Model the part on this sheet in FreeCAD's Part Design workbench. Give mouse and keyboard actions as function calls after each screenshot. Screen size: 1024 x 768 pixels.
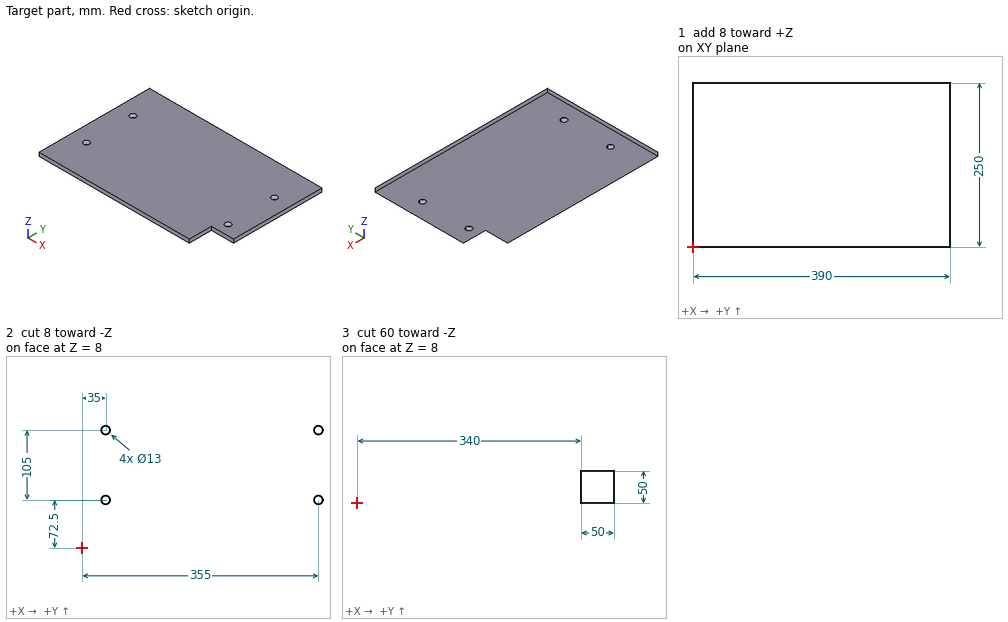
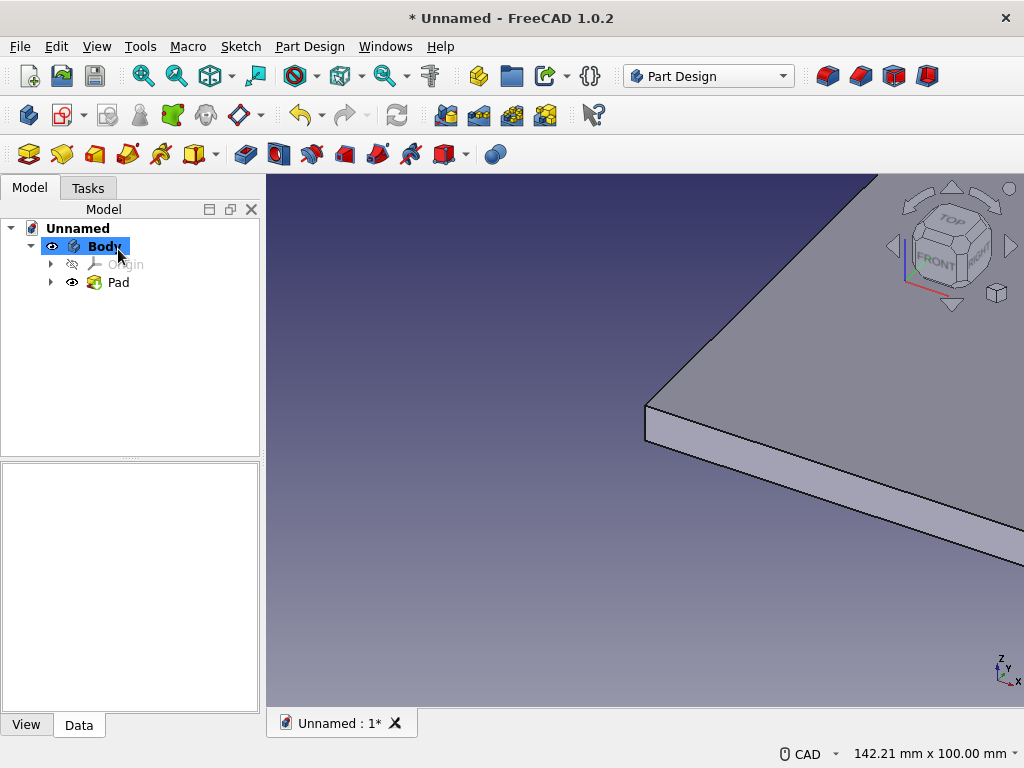
click(144, 76)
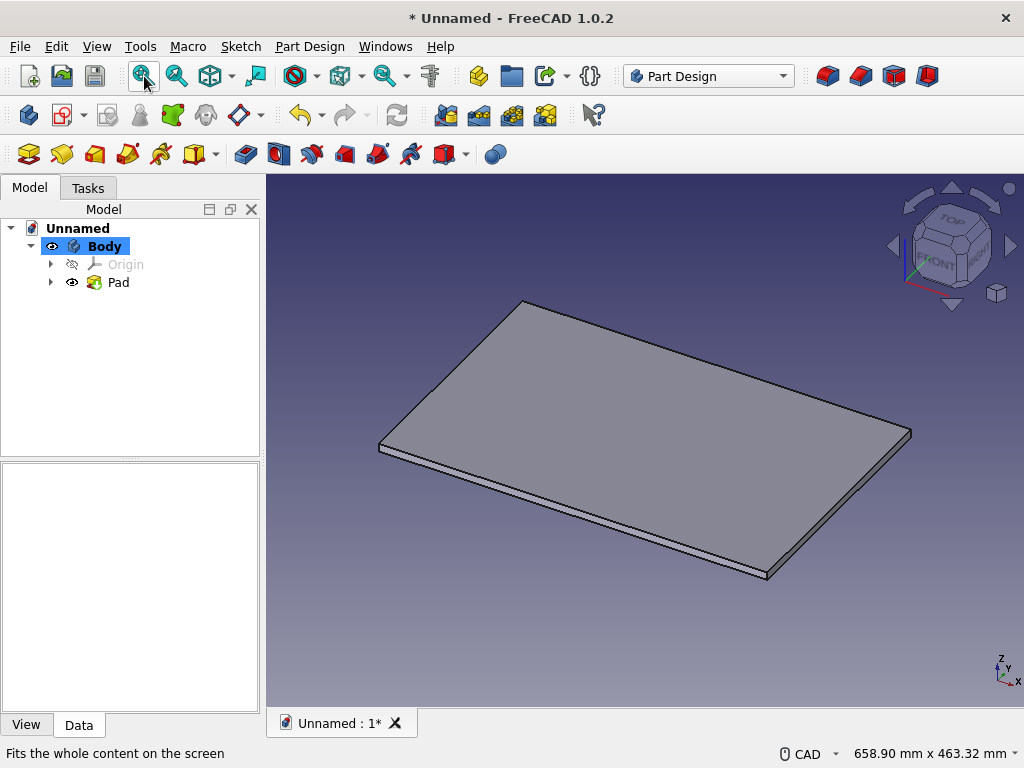
click(701, 454)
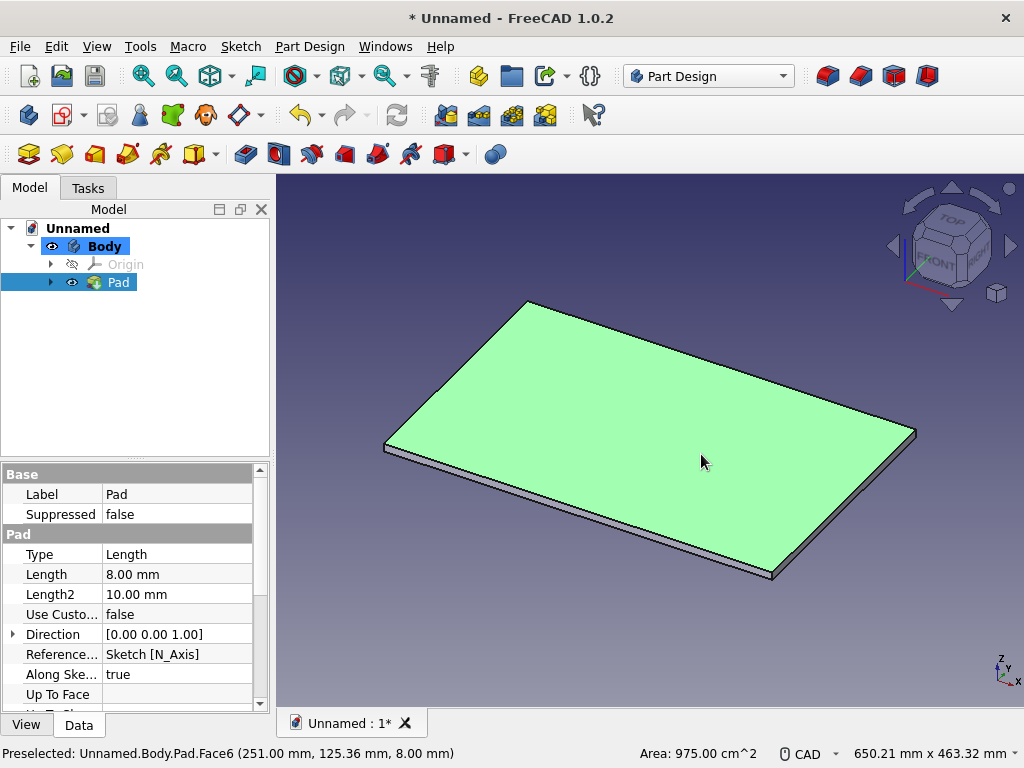
click(62, 116)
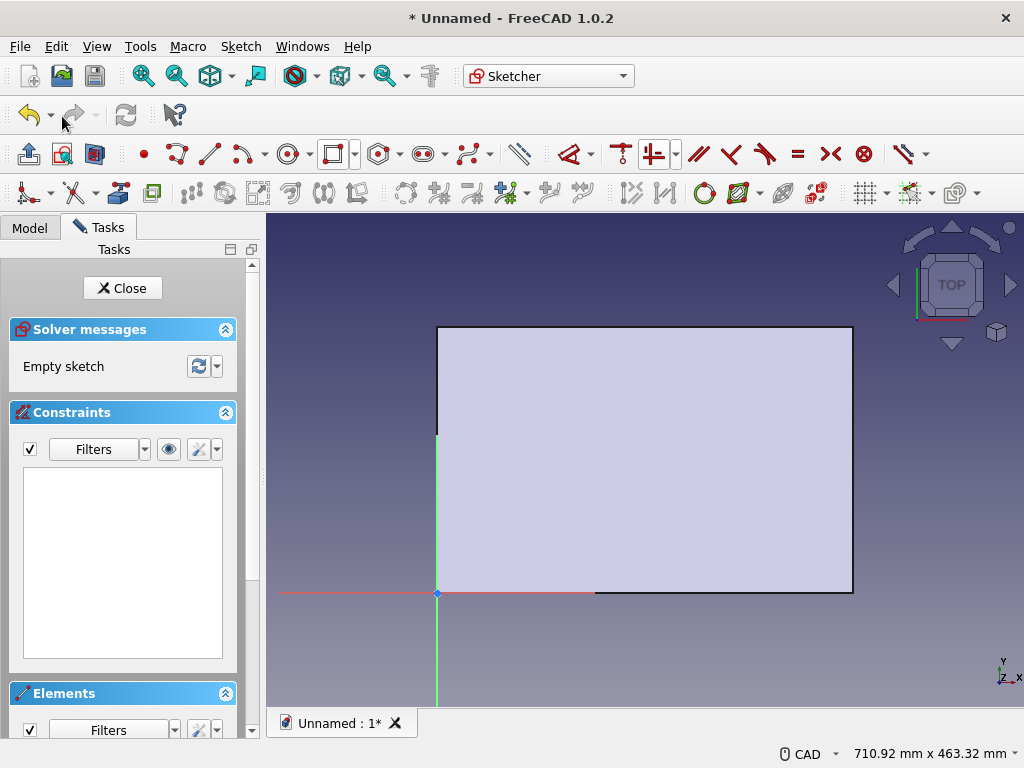
key(g)
key(c)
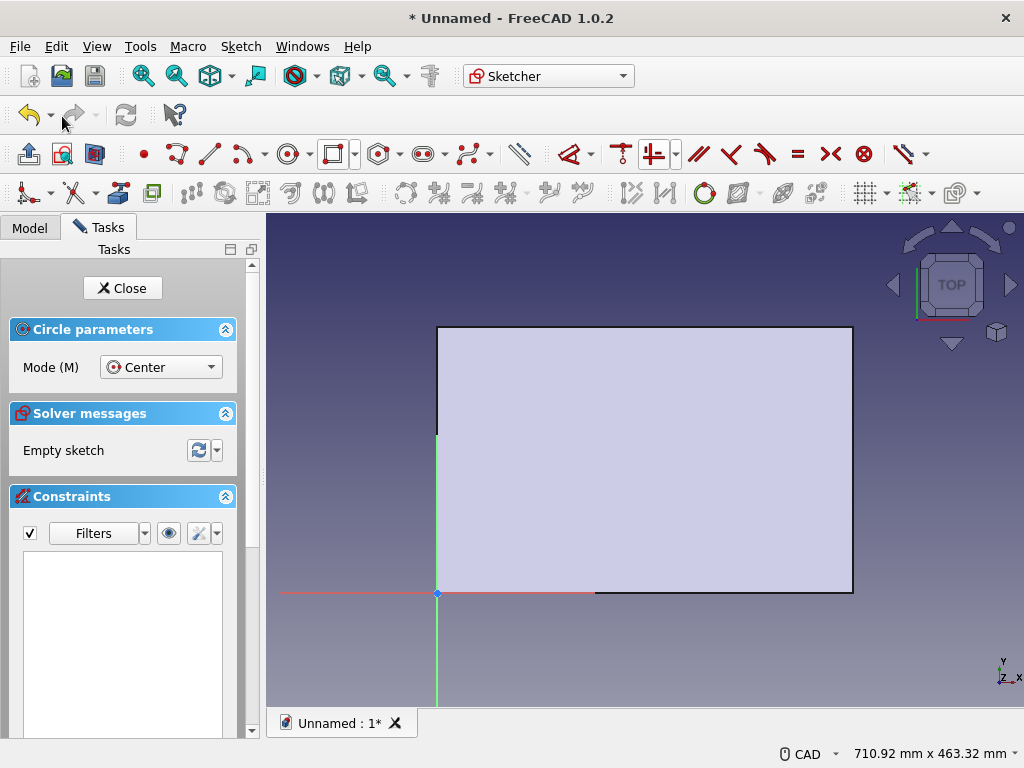
scroll(474, 404, up, 6)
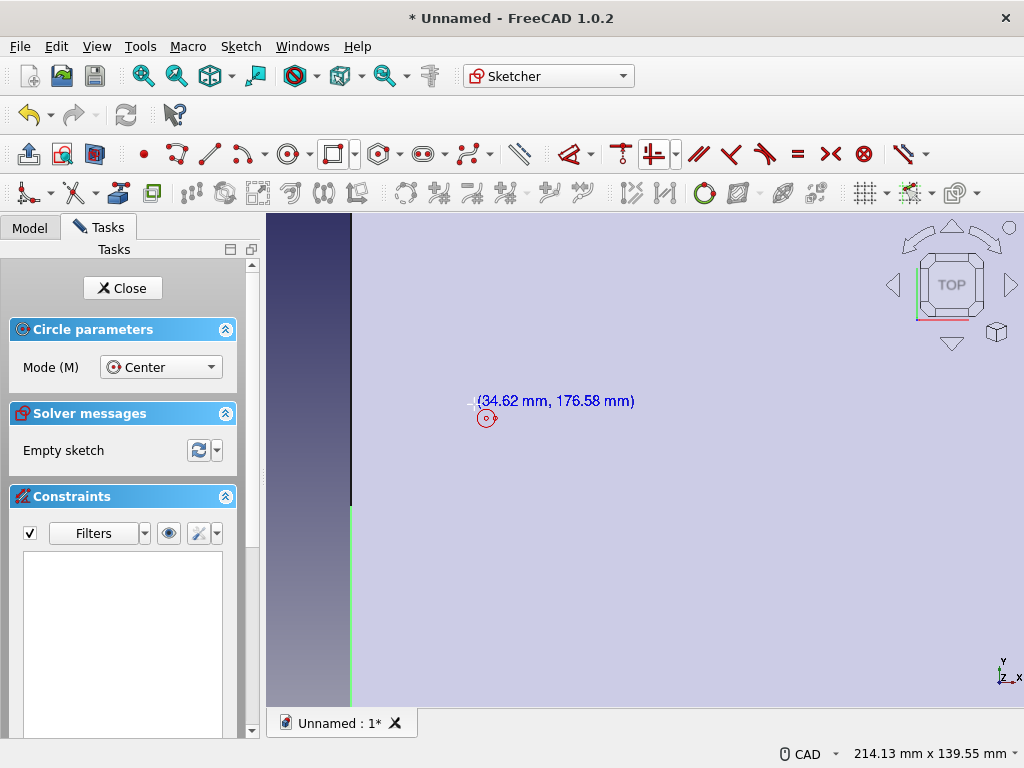
click(475, 403)
move(491, 387)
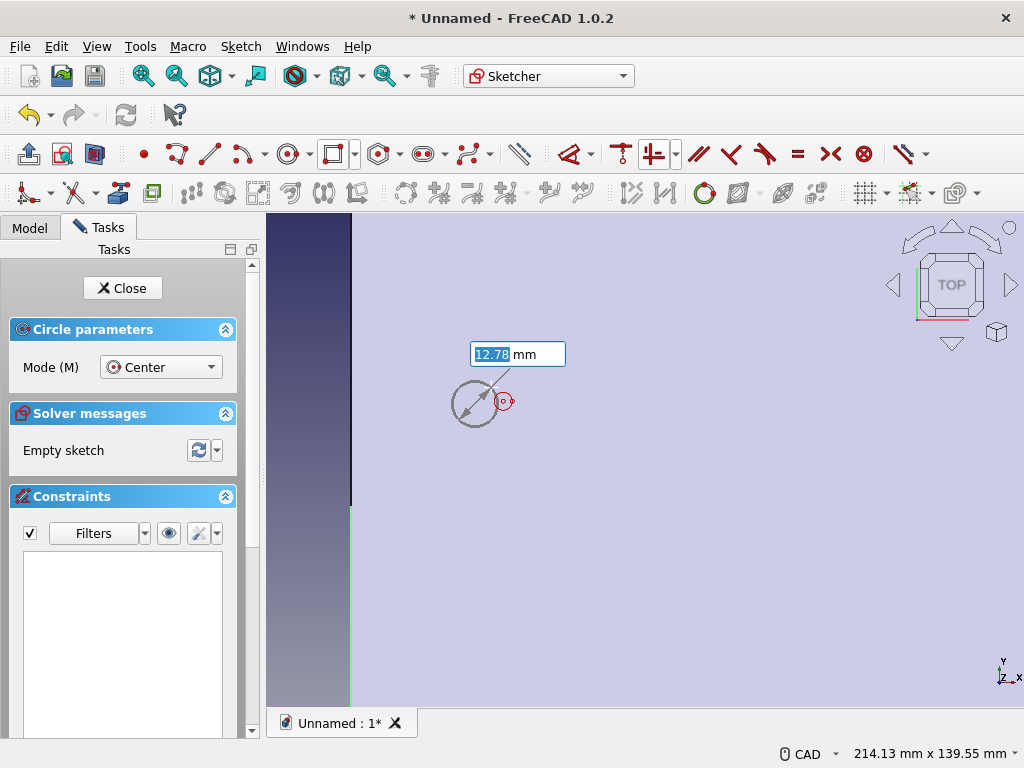
text(13)
key(Return)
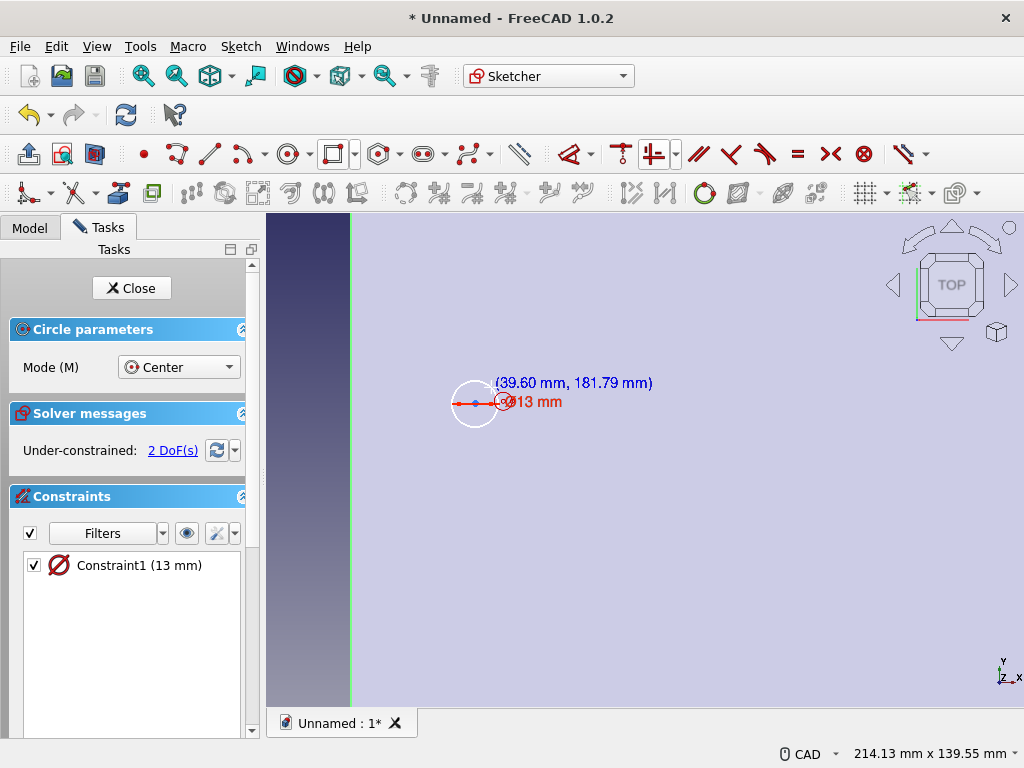
scroll(398, 354, down, 6)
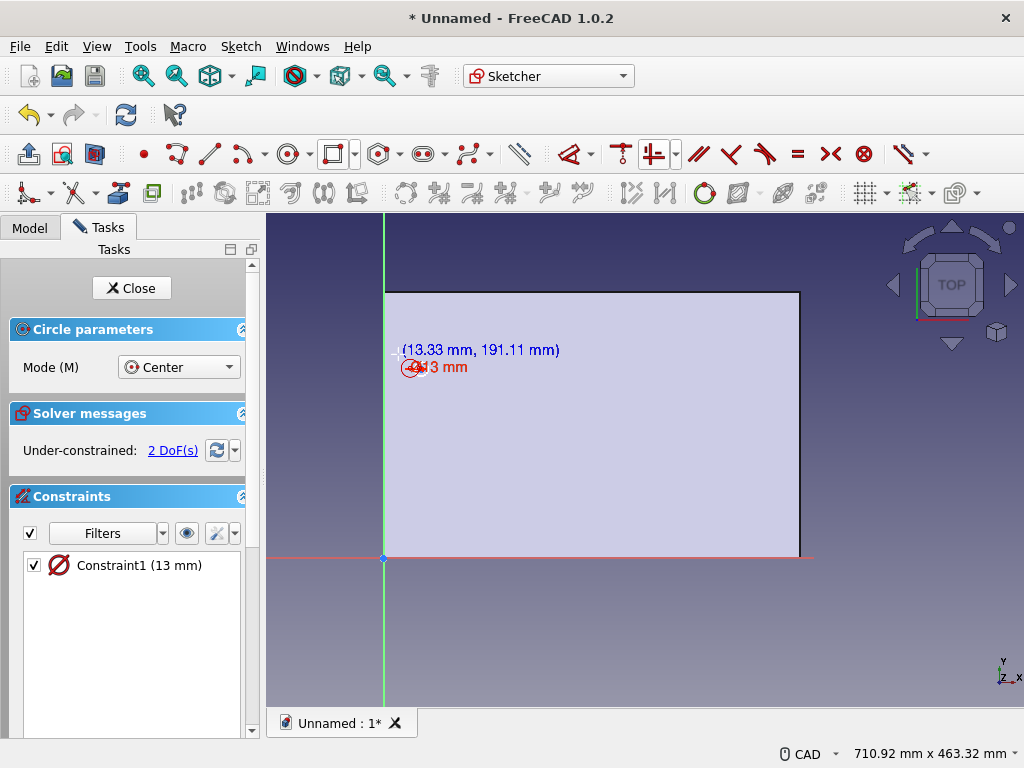
scroll(421, 481, up, 6)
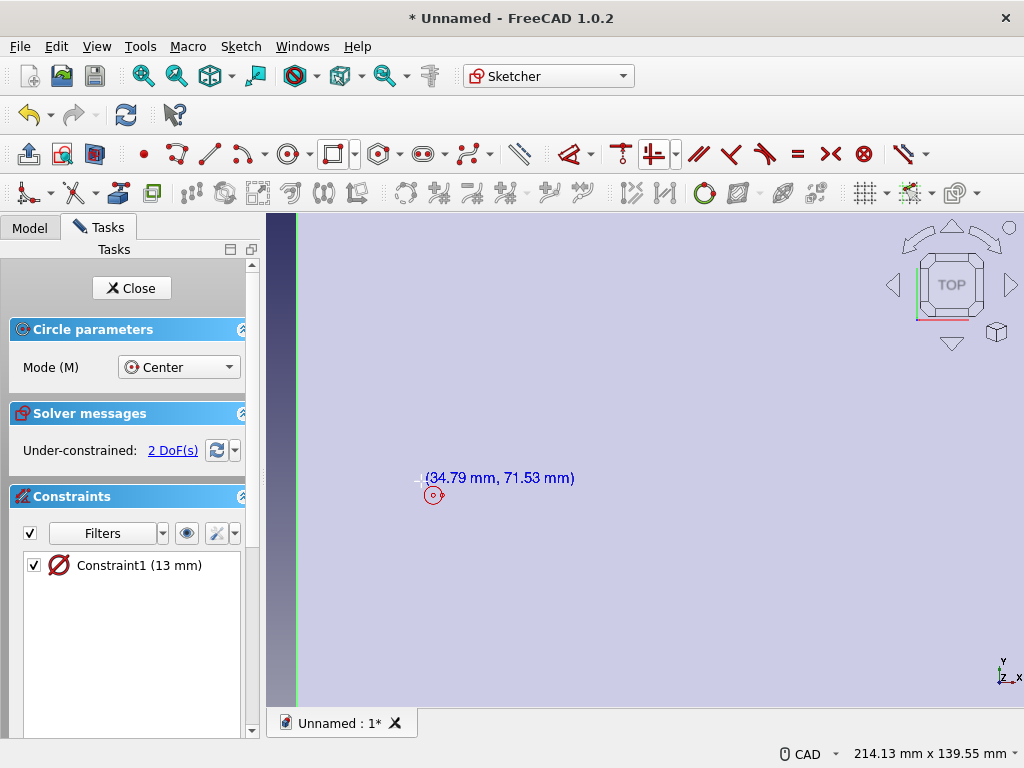
click(421, 480)
move(438, 463)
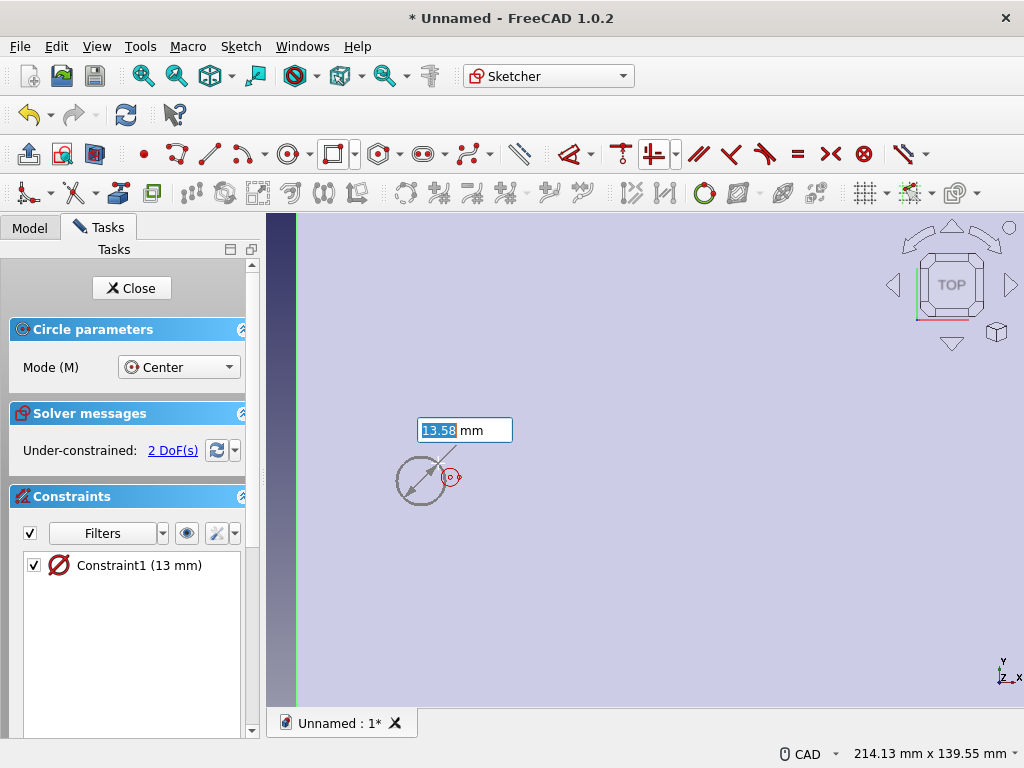
text(13)
key(Return)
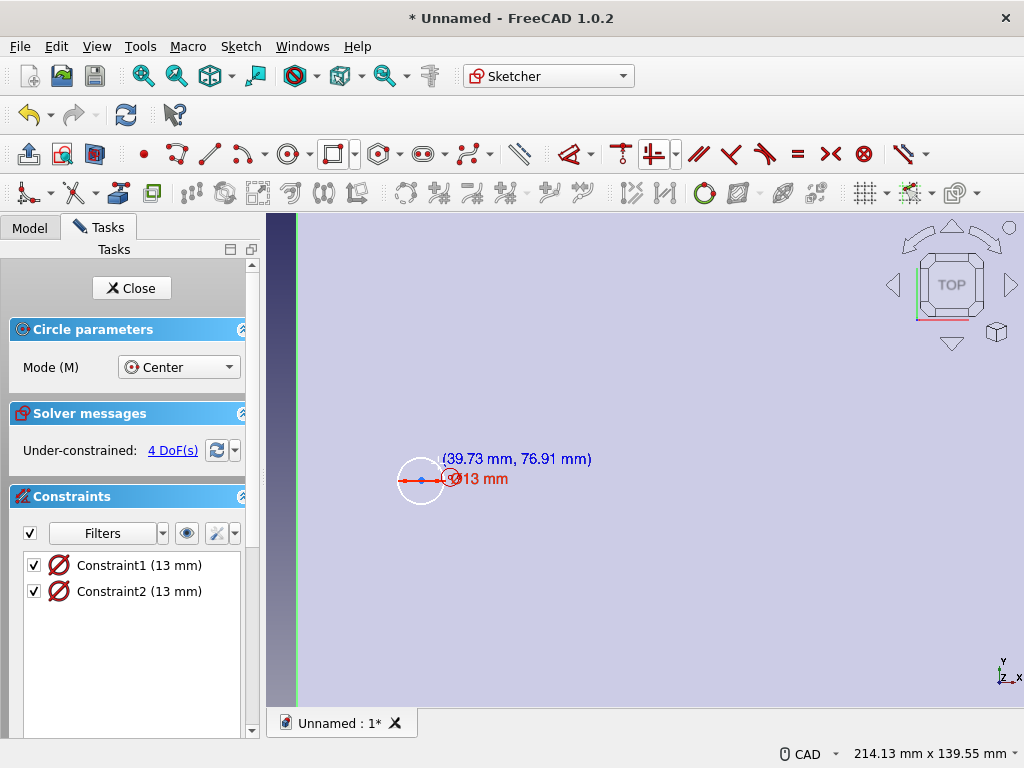
scroll(421, 481, down, 6)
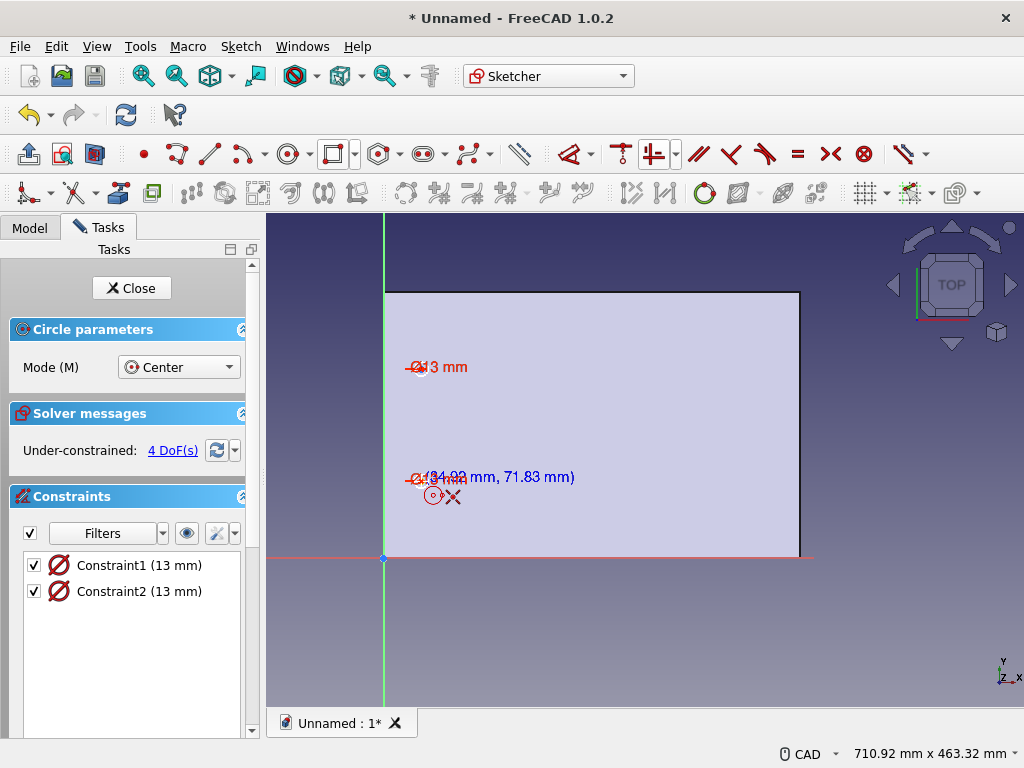
scroll(762, 481, up, 6)